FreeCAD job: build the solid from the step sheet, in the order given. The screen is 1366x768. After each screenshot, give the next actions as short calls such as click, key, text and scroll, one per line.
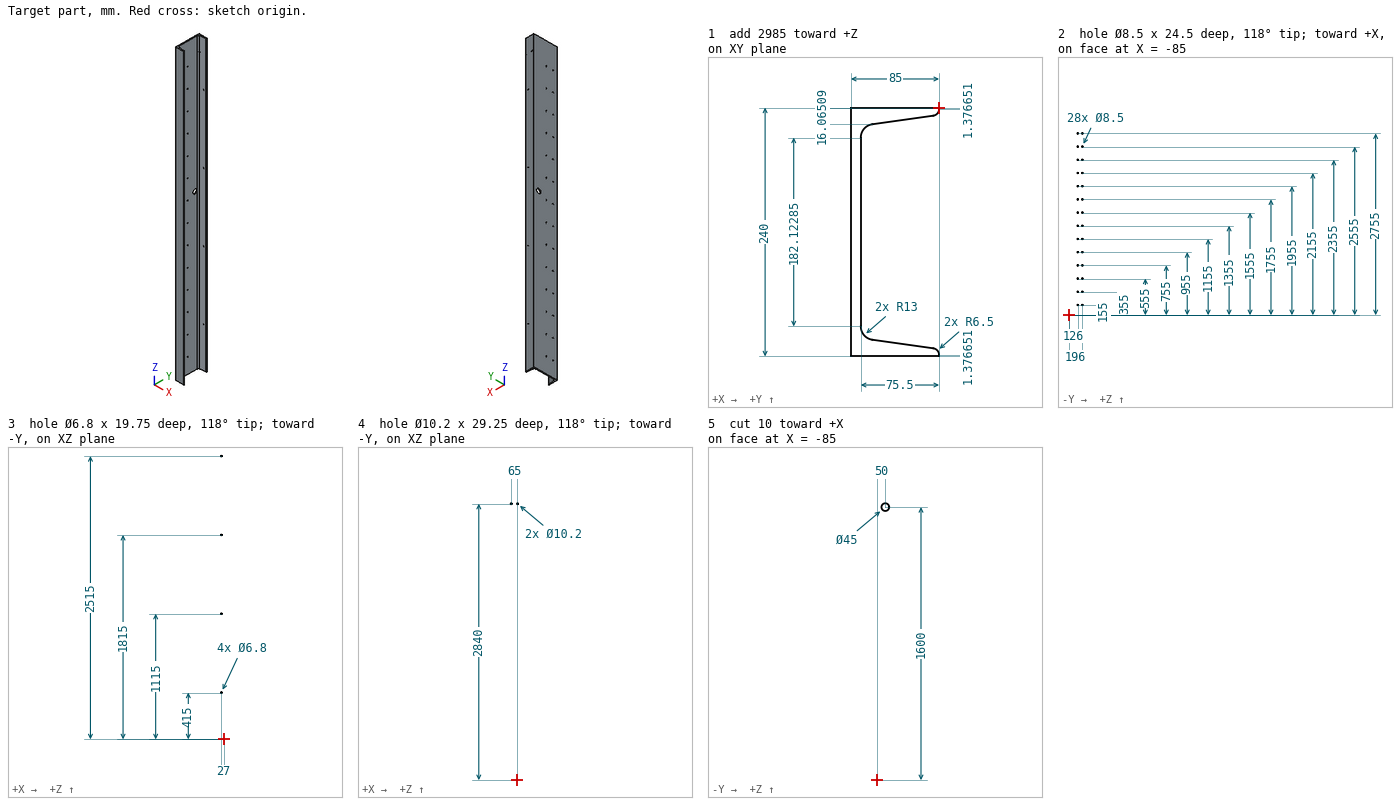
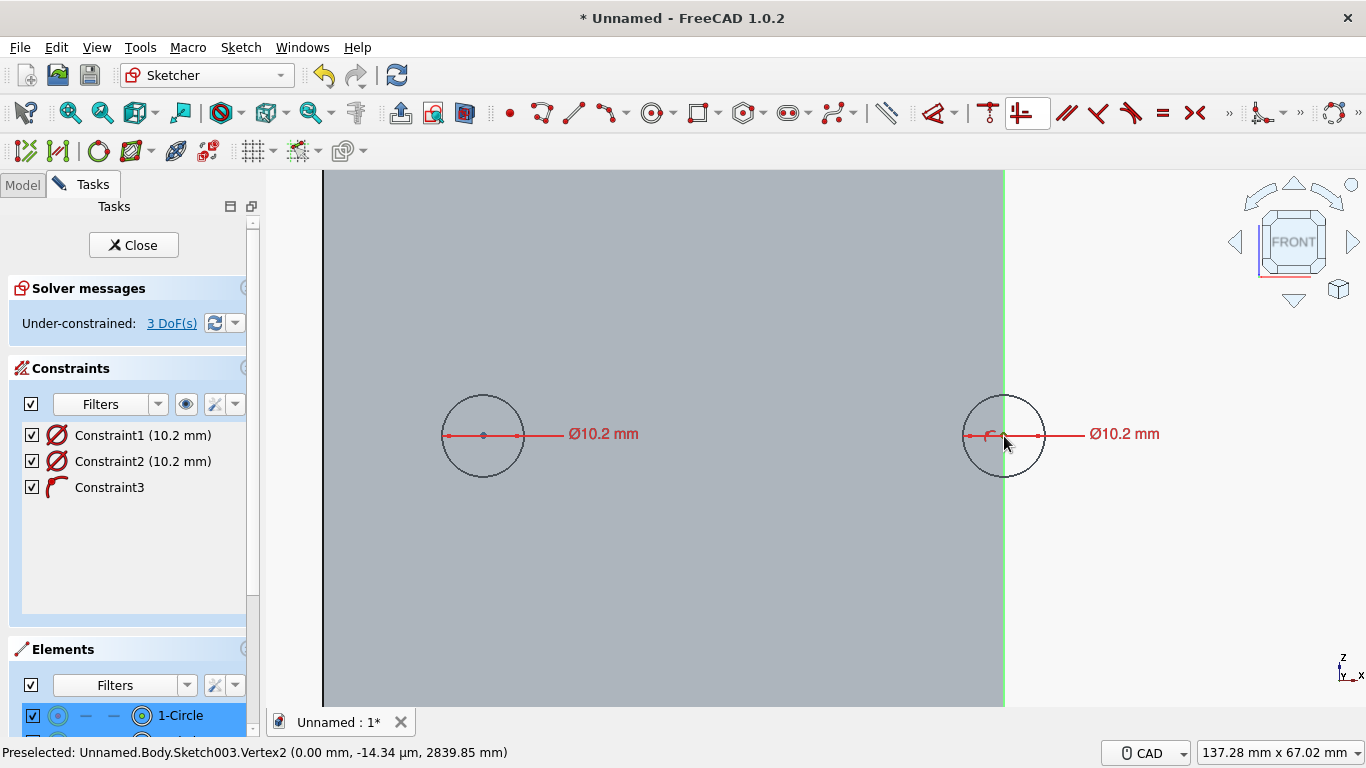
key(h)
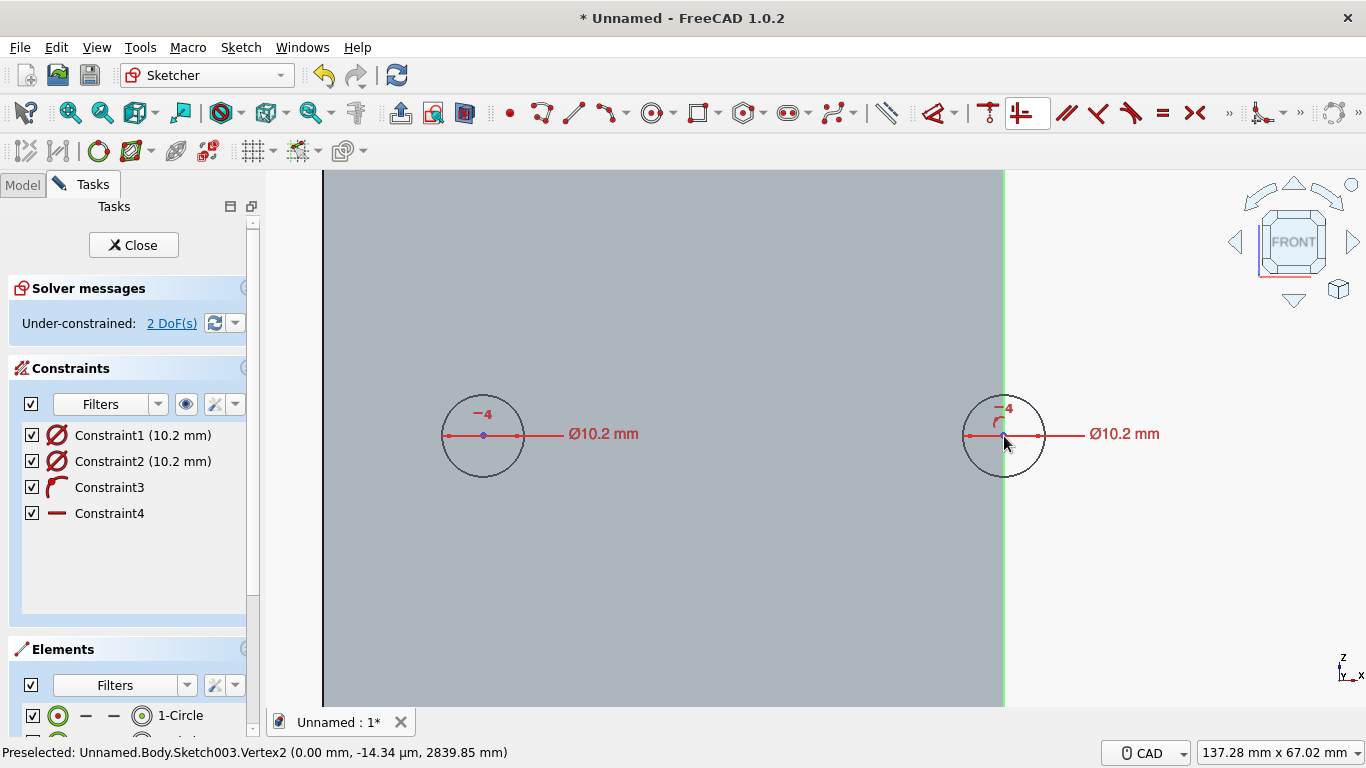
click(934, 114)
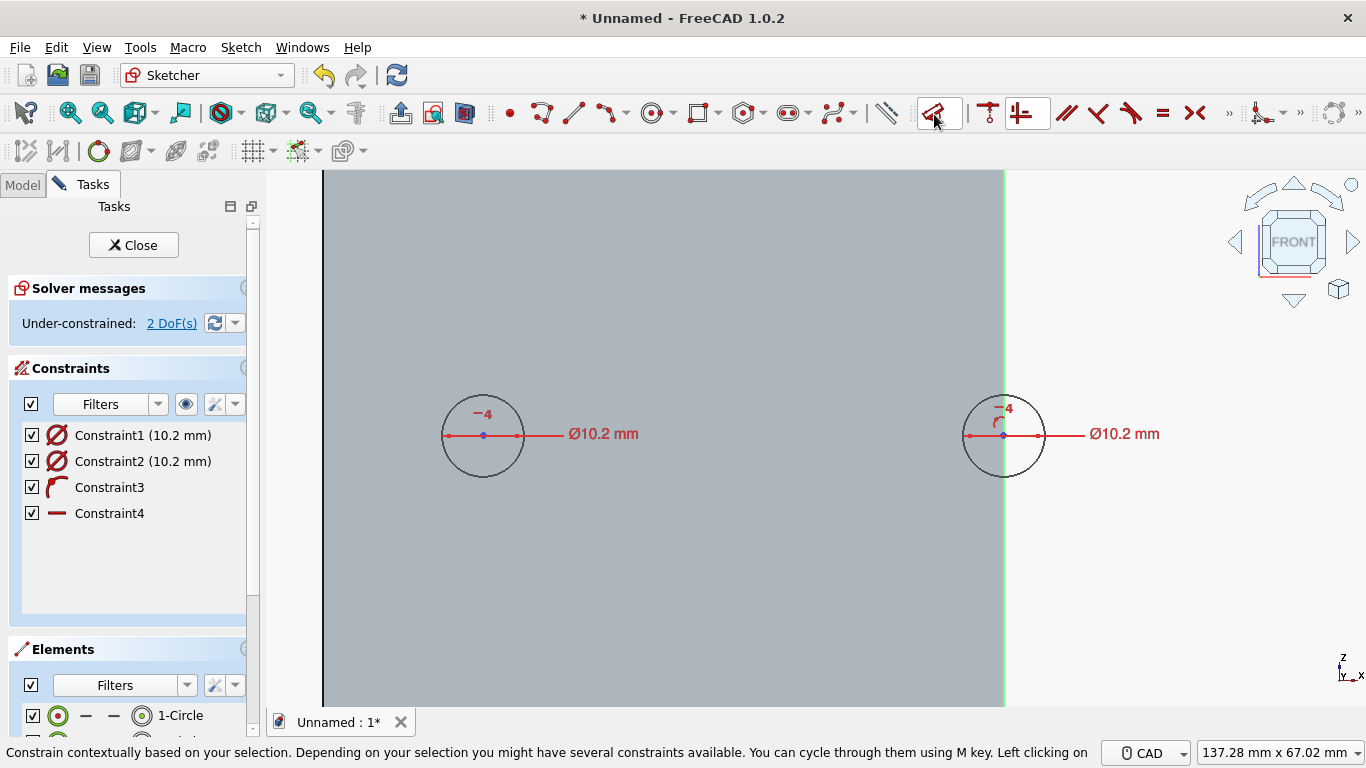
click(483, 436)
click(743, 402)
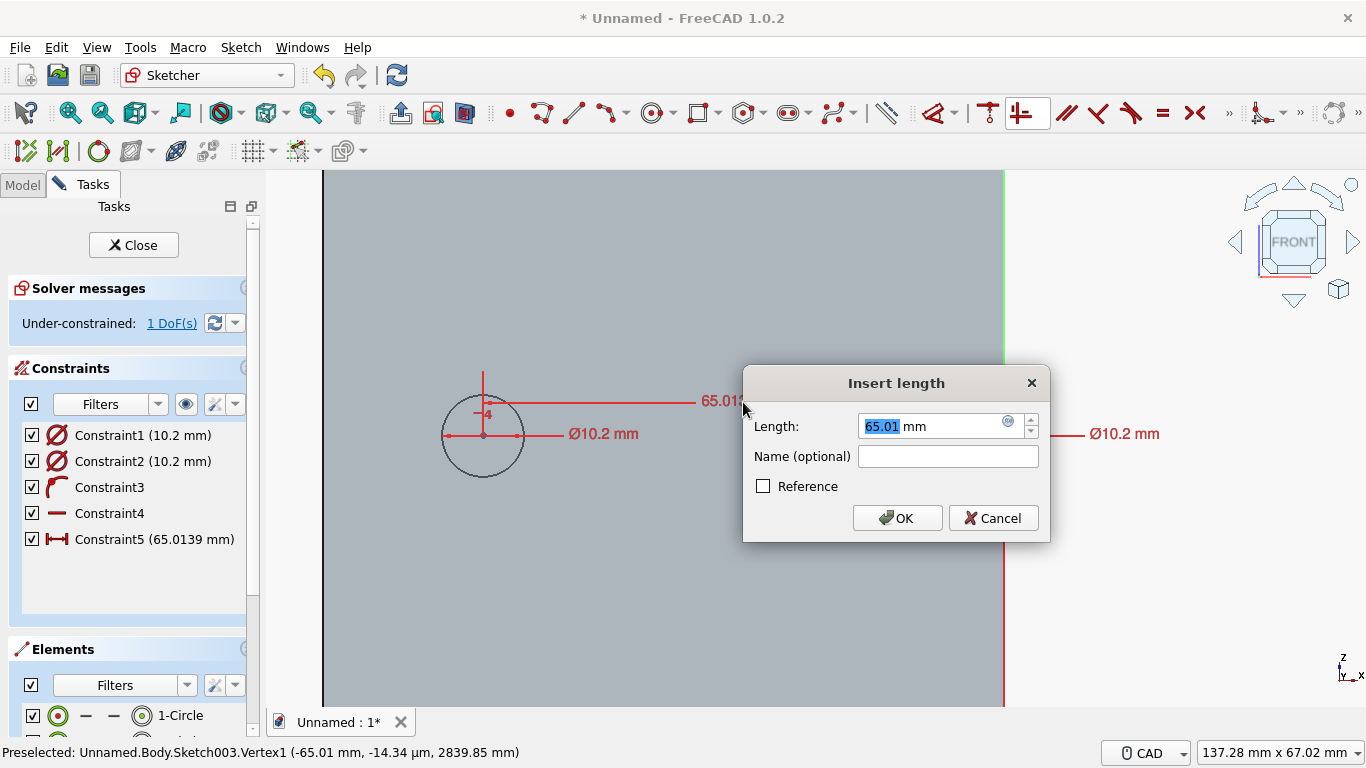
text(65)
key(Return)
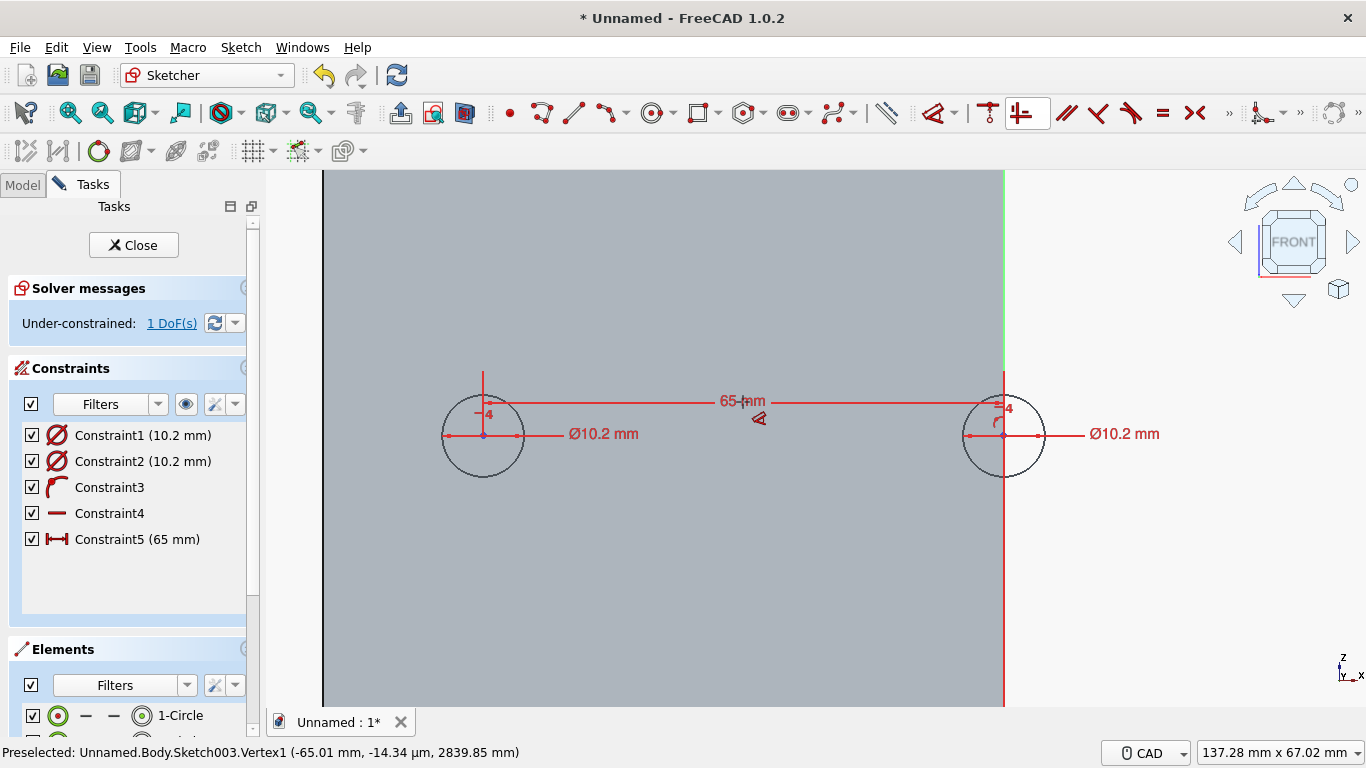
click(483, 436)
click(1038, 557)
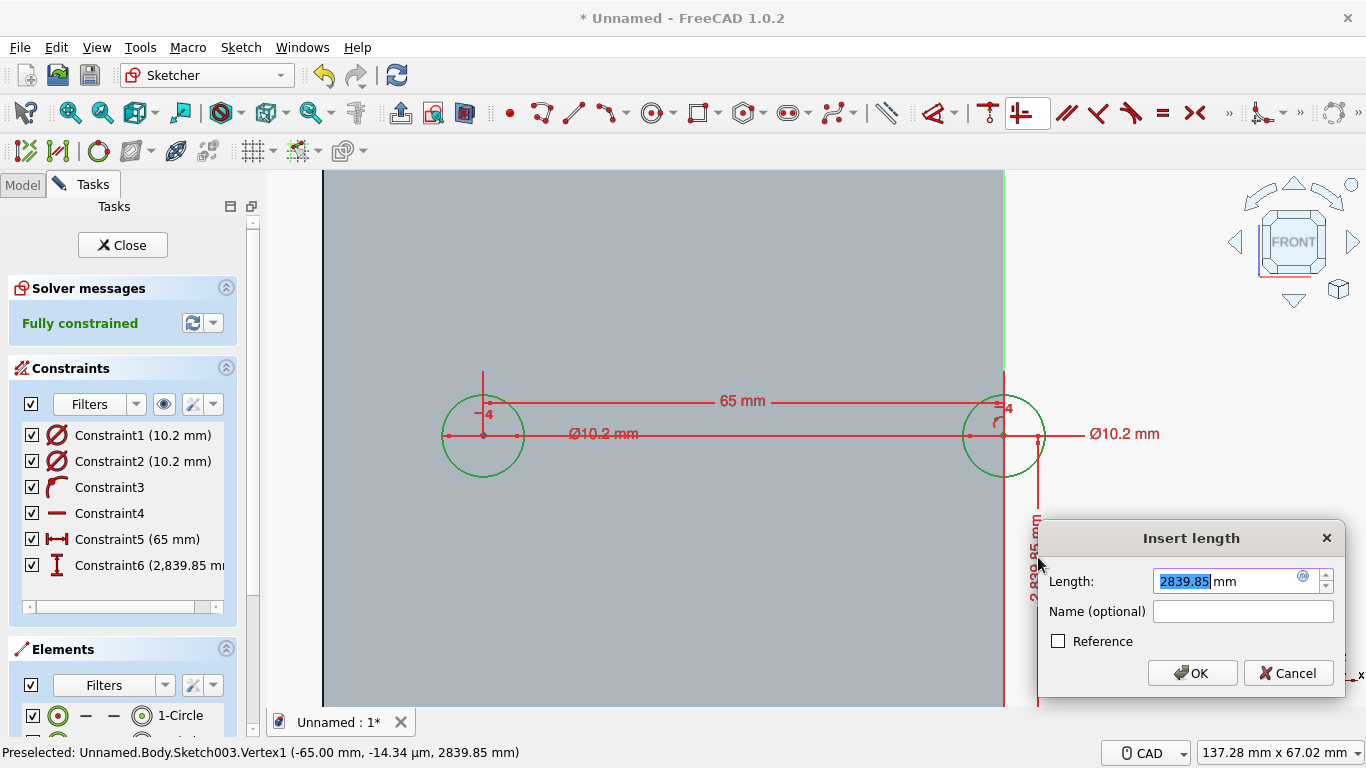
text(2840)
key(Return)
key(Escape)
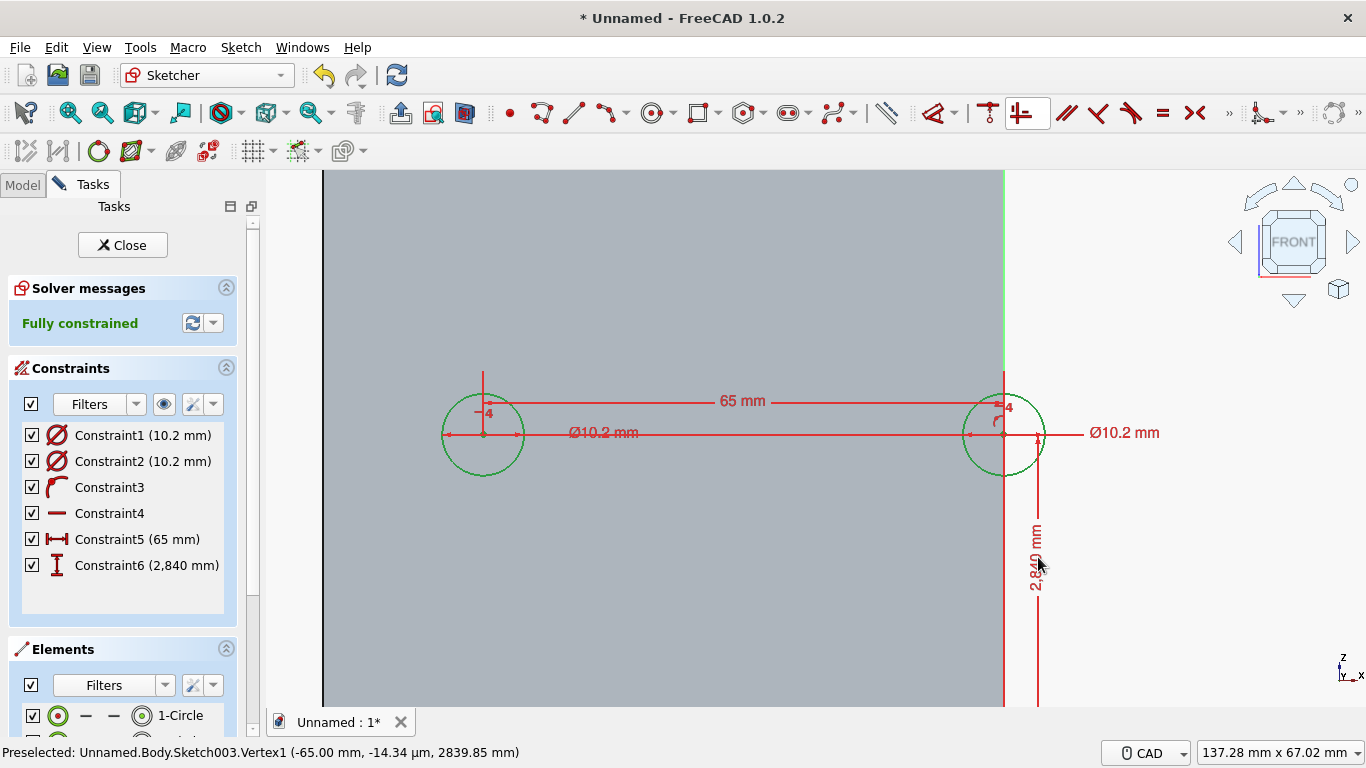
click(123, 245)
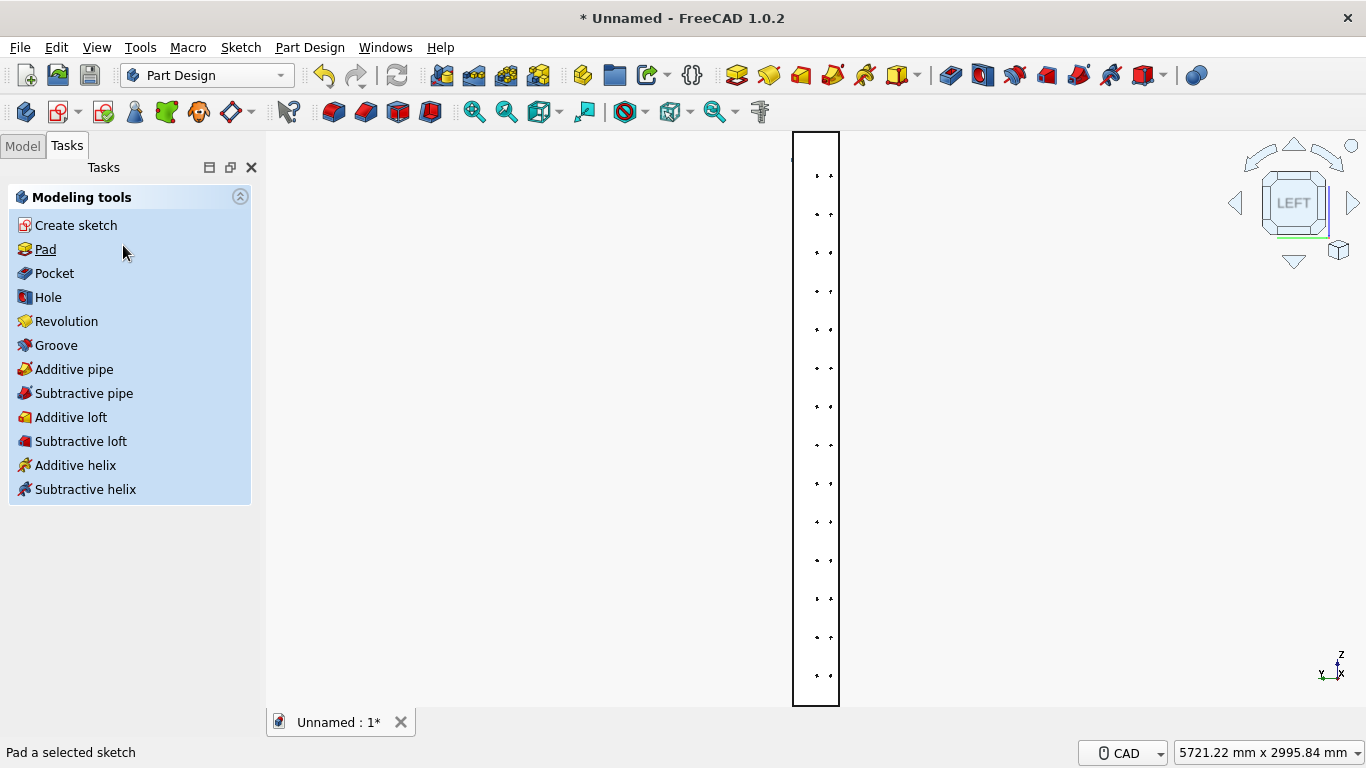
click(984, 76)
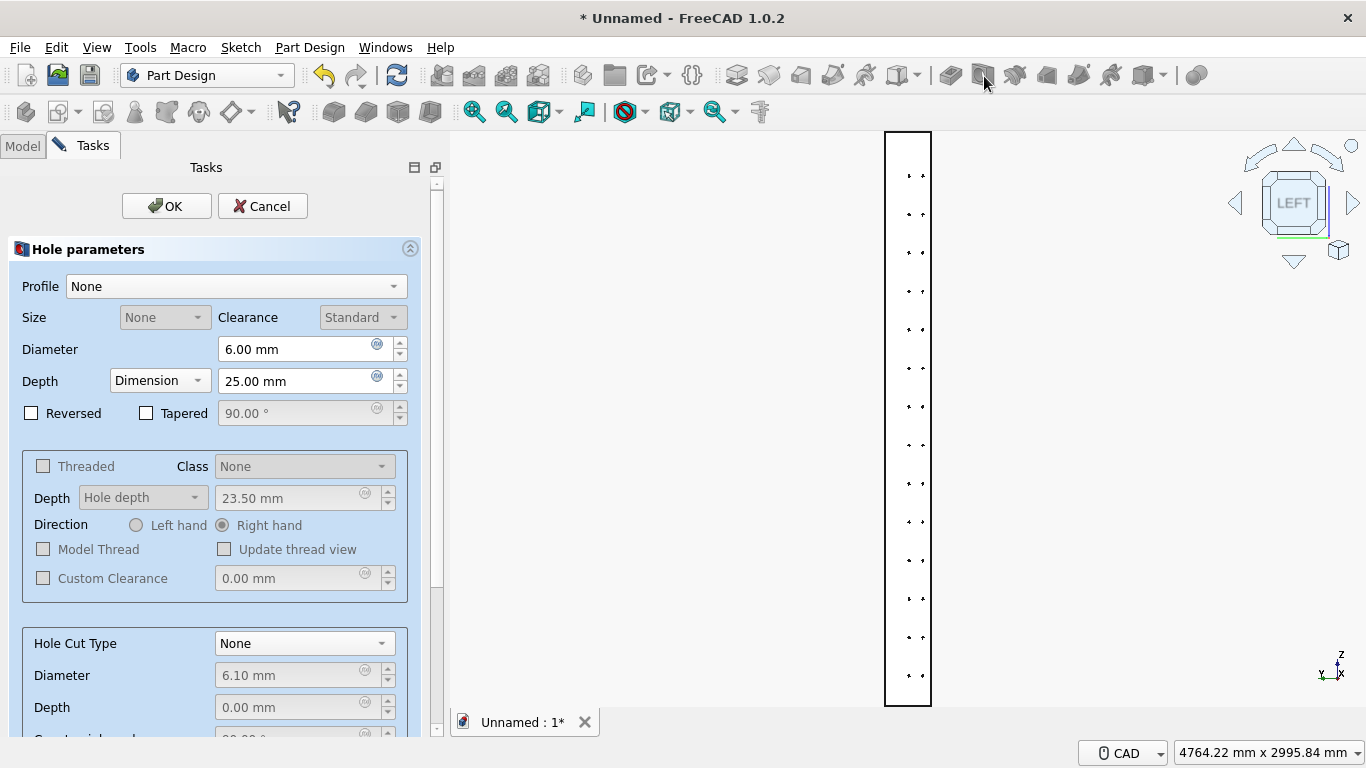
triple_click(305, 349)